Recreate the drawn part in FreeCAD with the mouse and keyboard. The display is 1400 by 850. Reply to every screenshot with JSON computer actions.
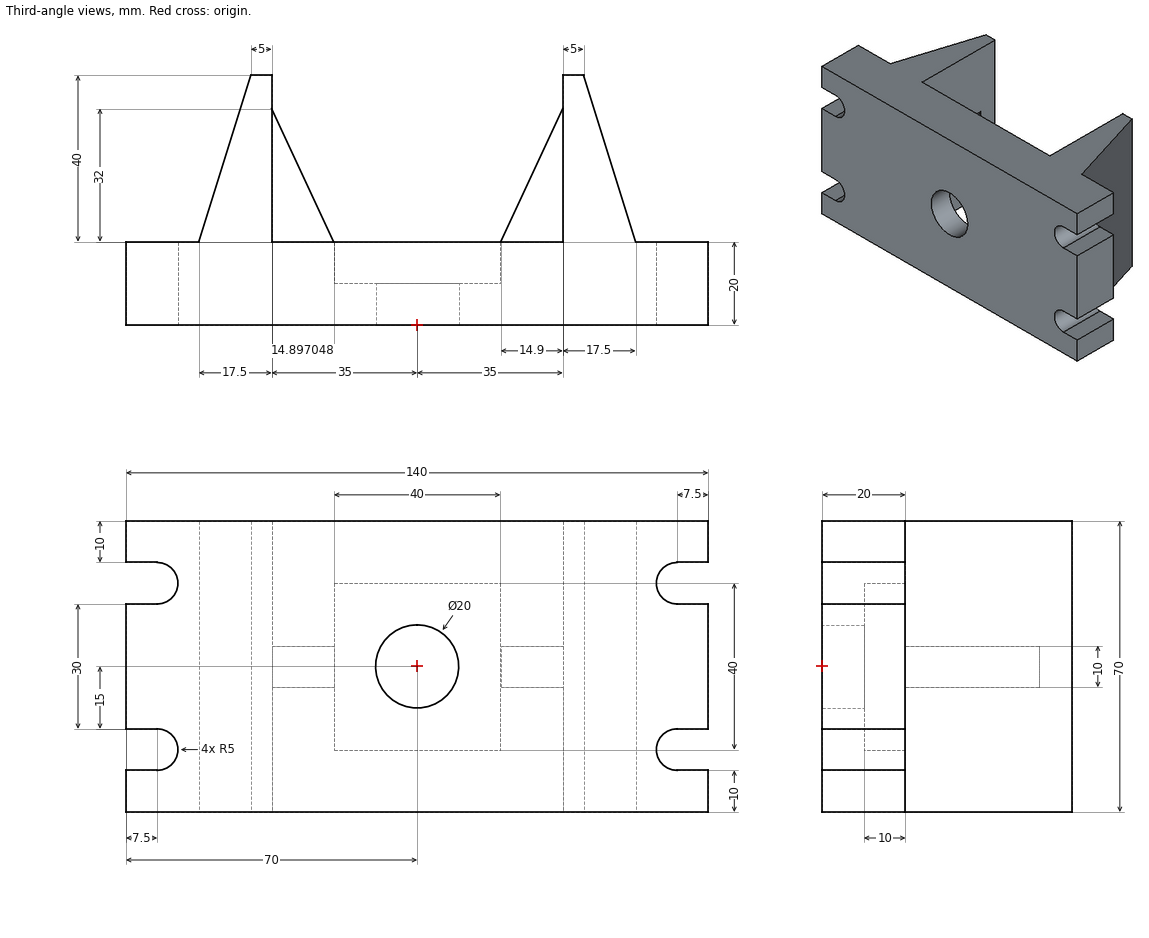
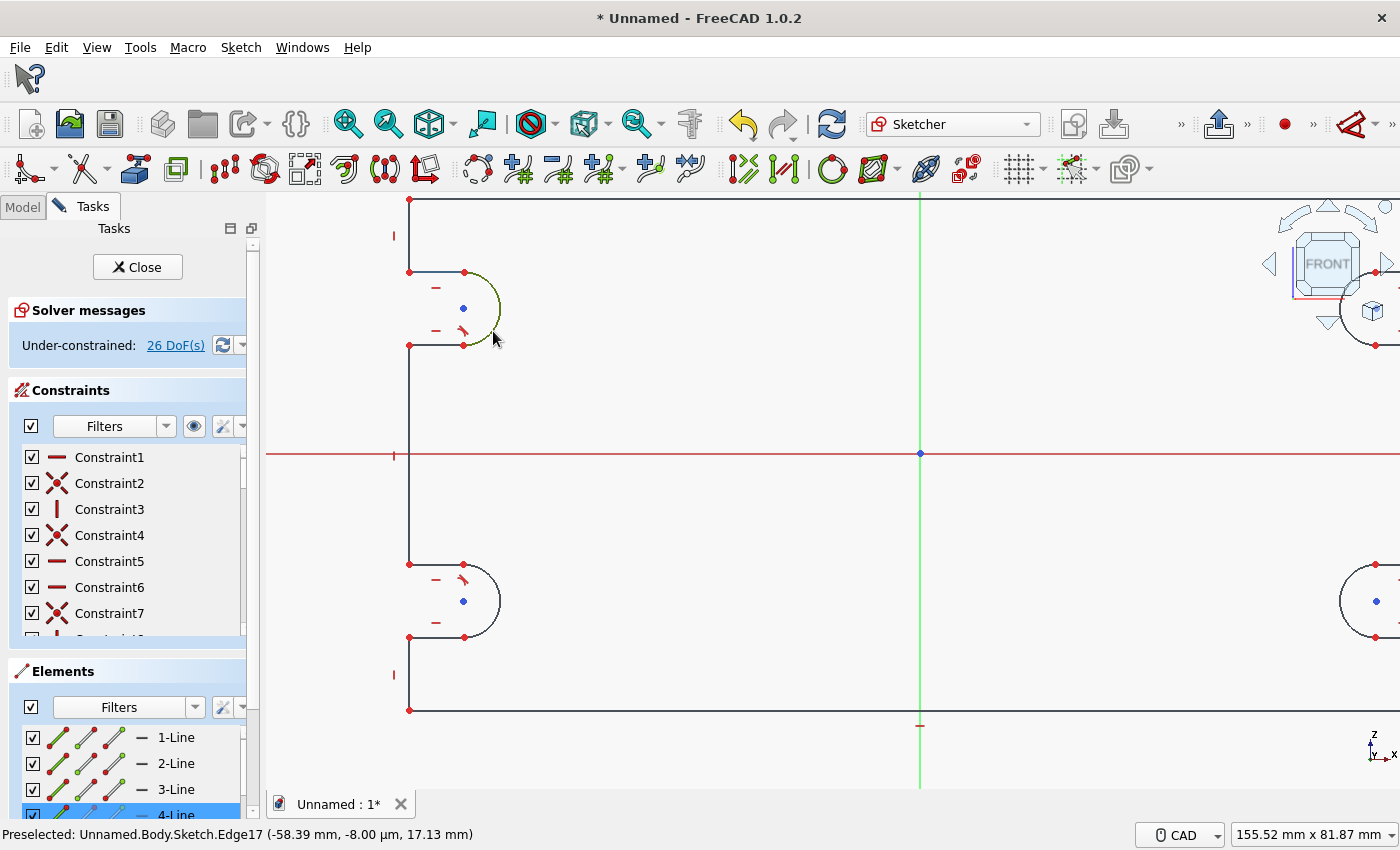
{"action": "key", "text": "t"}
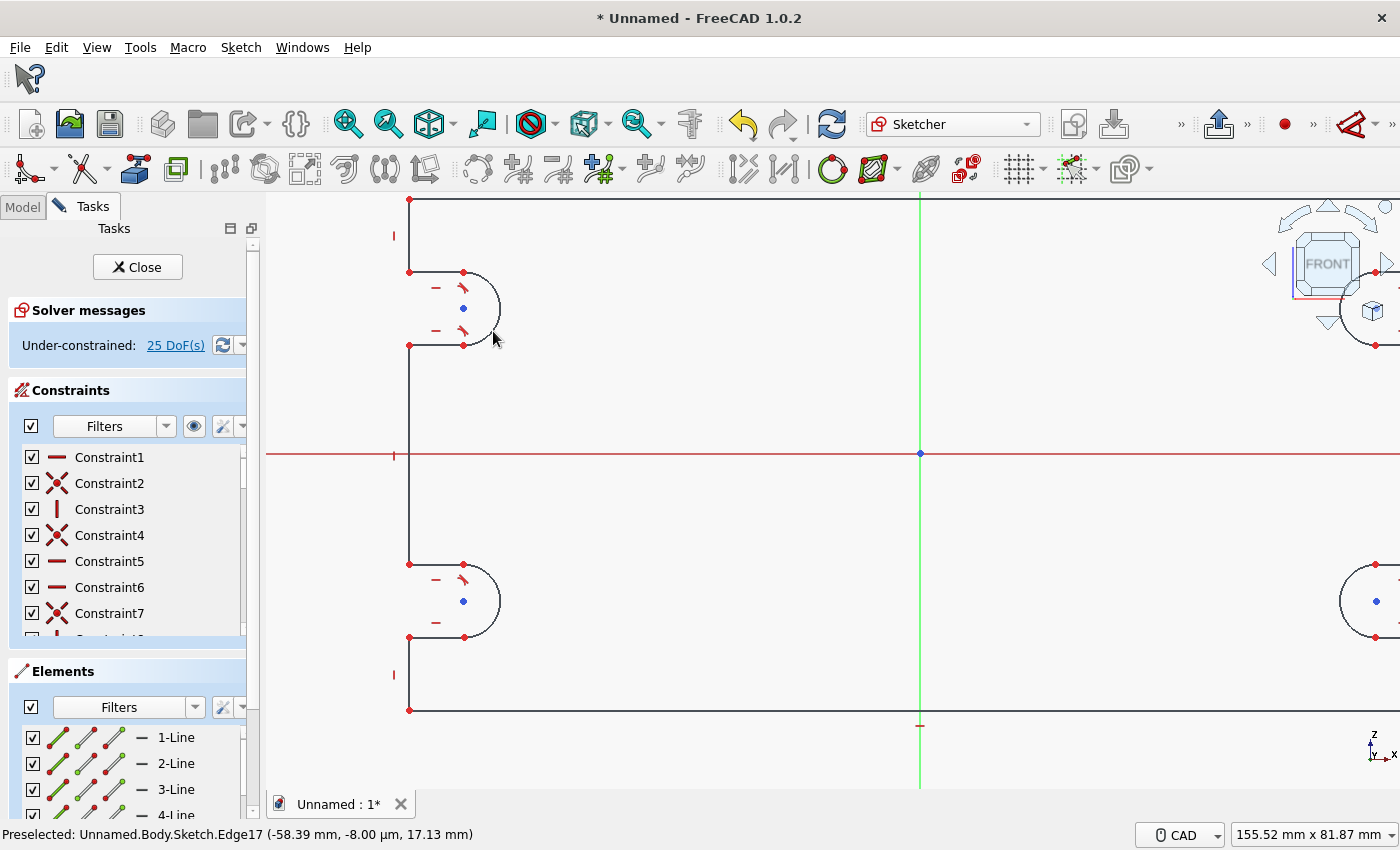
{"action": "scroll", "coordinate": [448, 566], "scroll_direction": "down", "scroll_amount": 2}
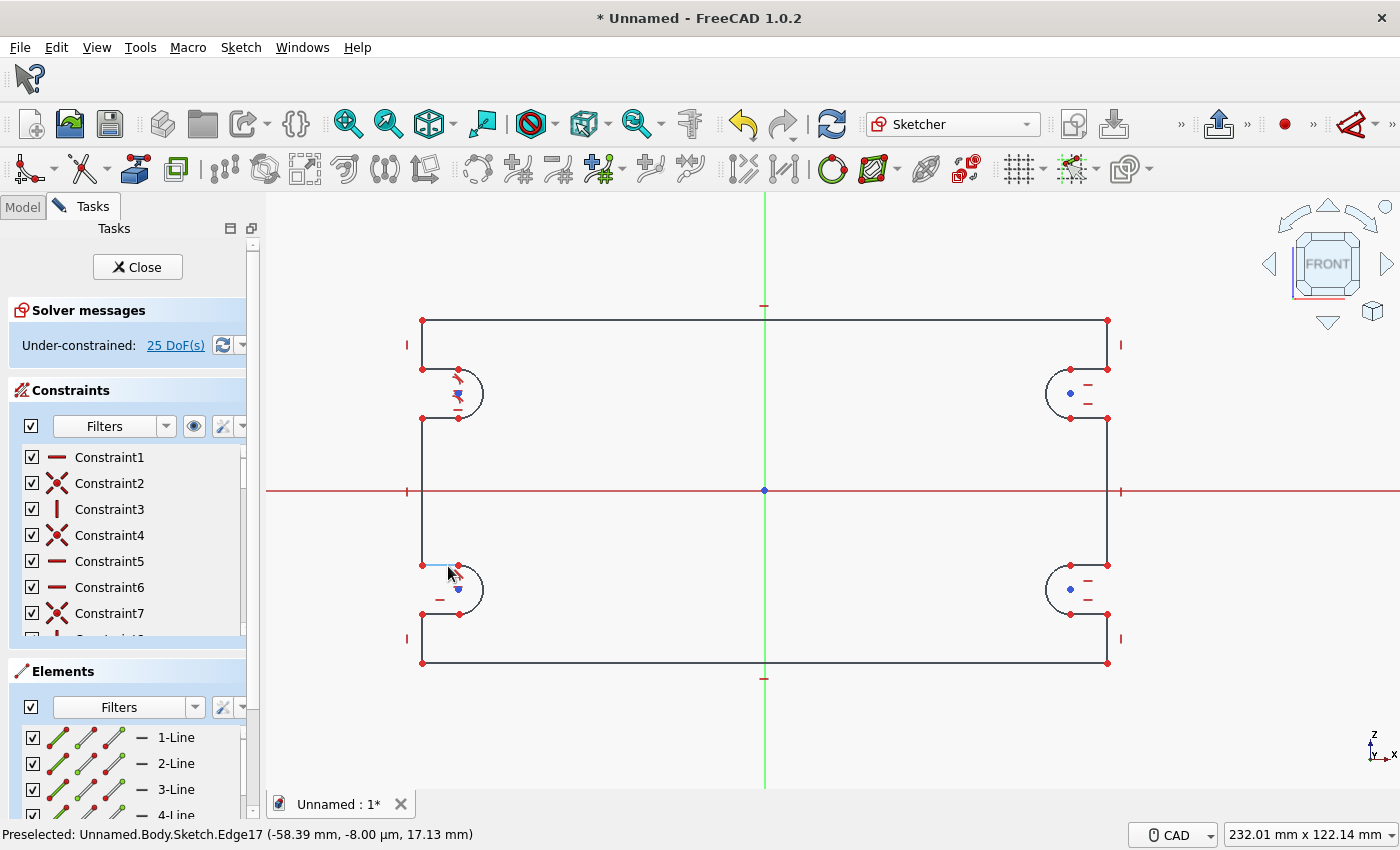
{"action": "scroll", "coordinate": [1096, 369], "scroll_direction": "up", "scroll_amount": 2}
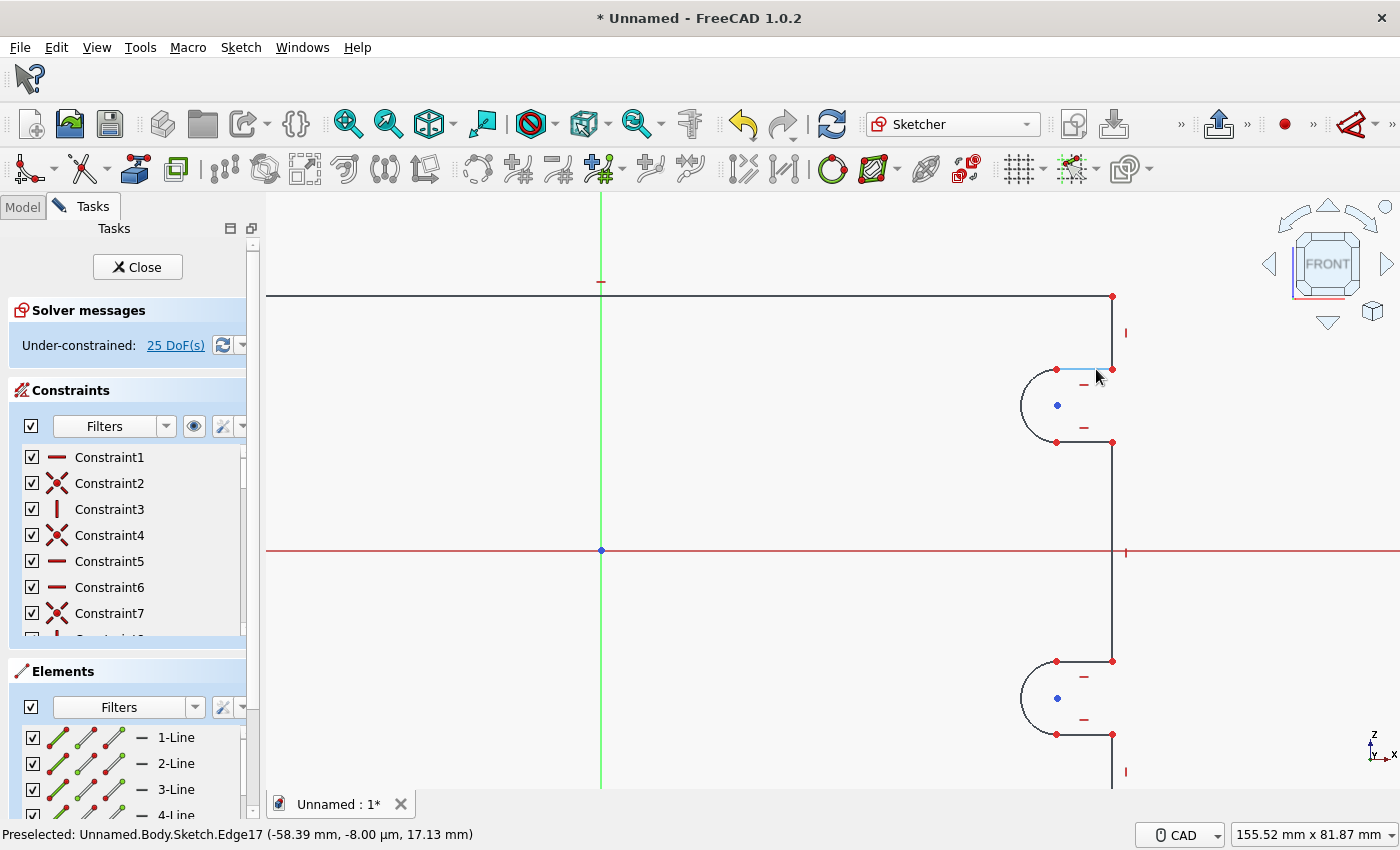
{"action": "left_click", "coordinate": [1095, 369]}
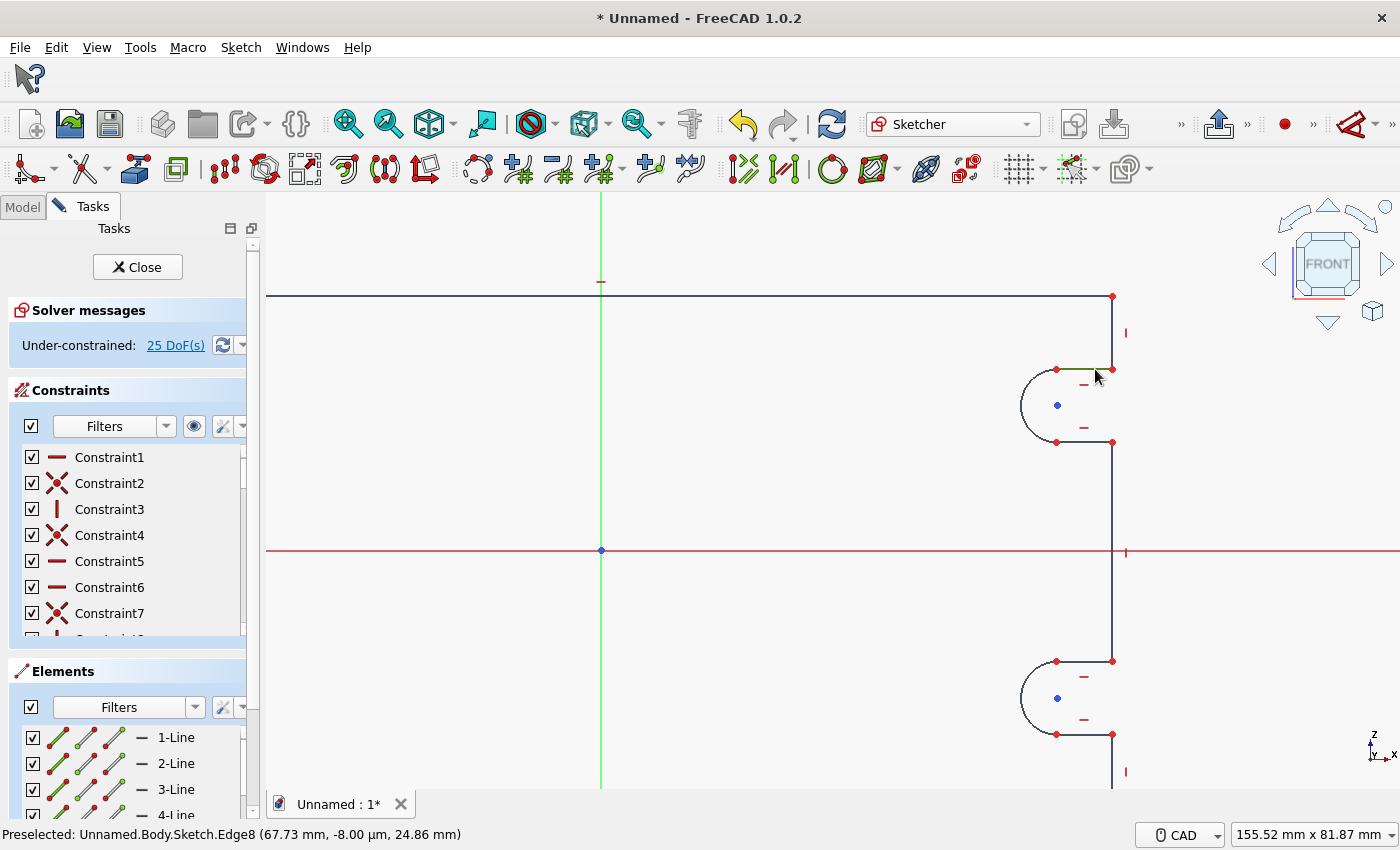
{"action": "left_click", "coordinate": [1028, 385]}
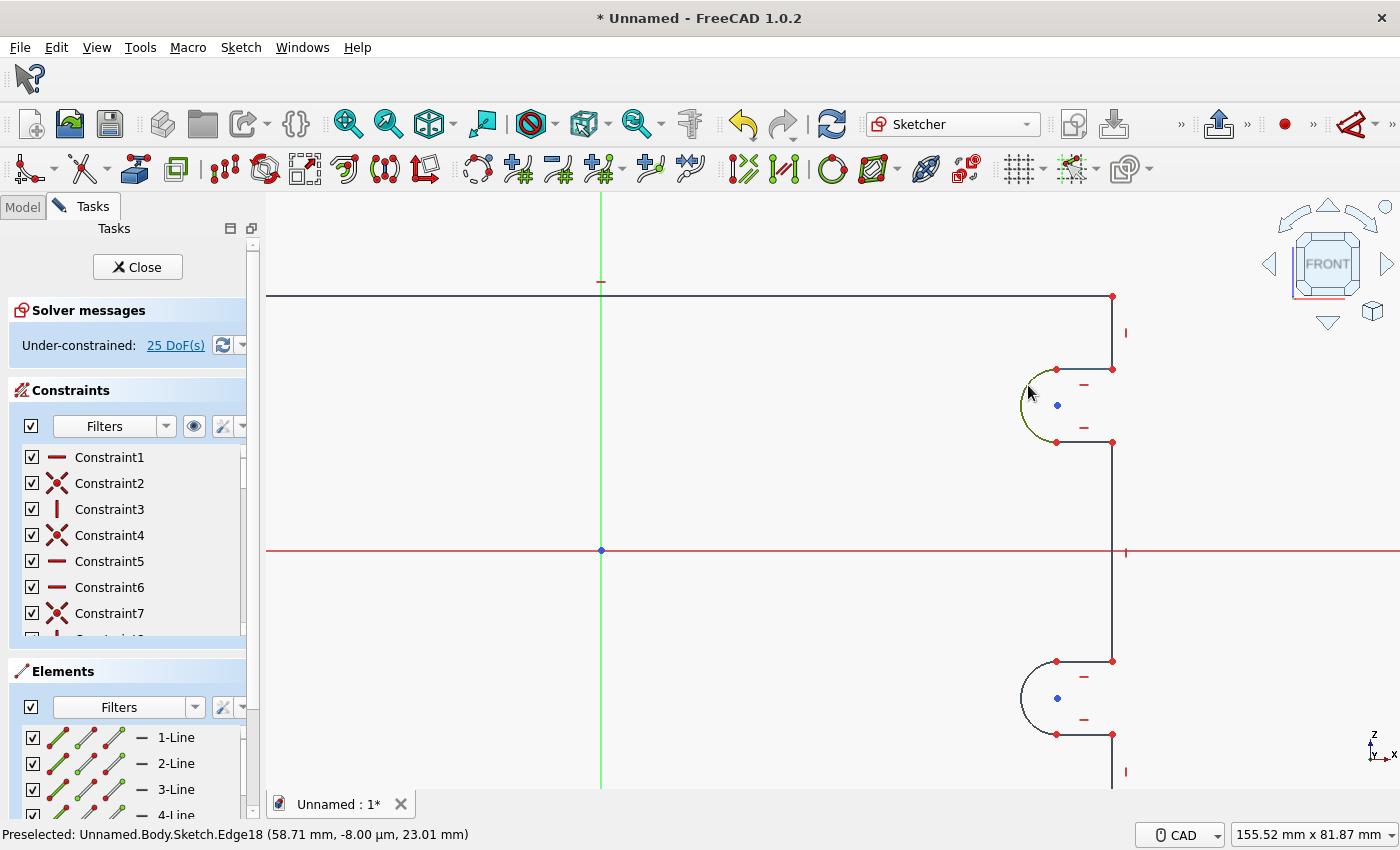
{"action": "key", "text": "t"}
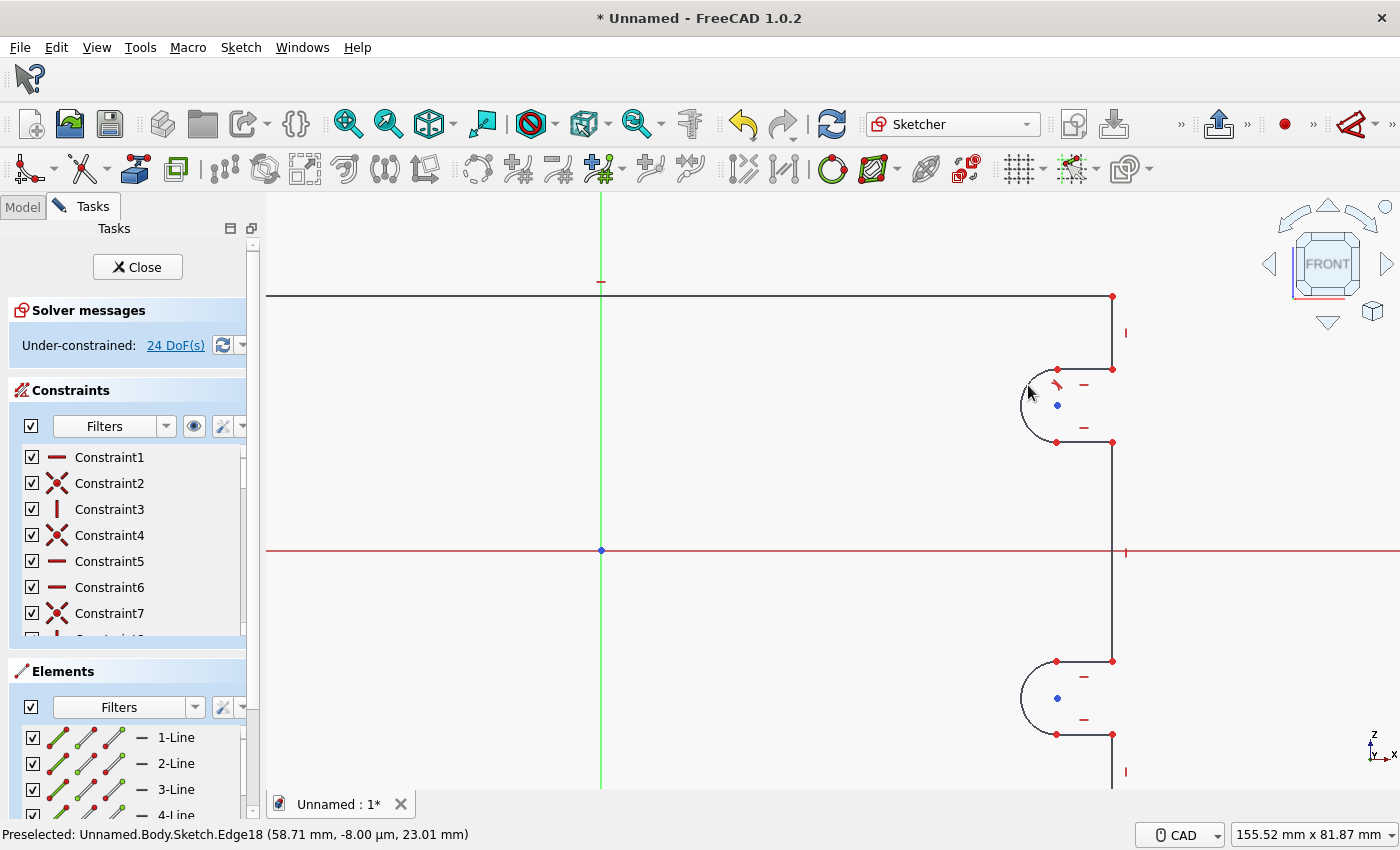
{"action": "left_click", "coordinate": [1073, 442]}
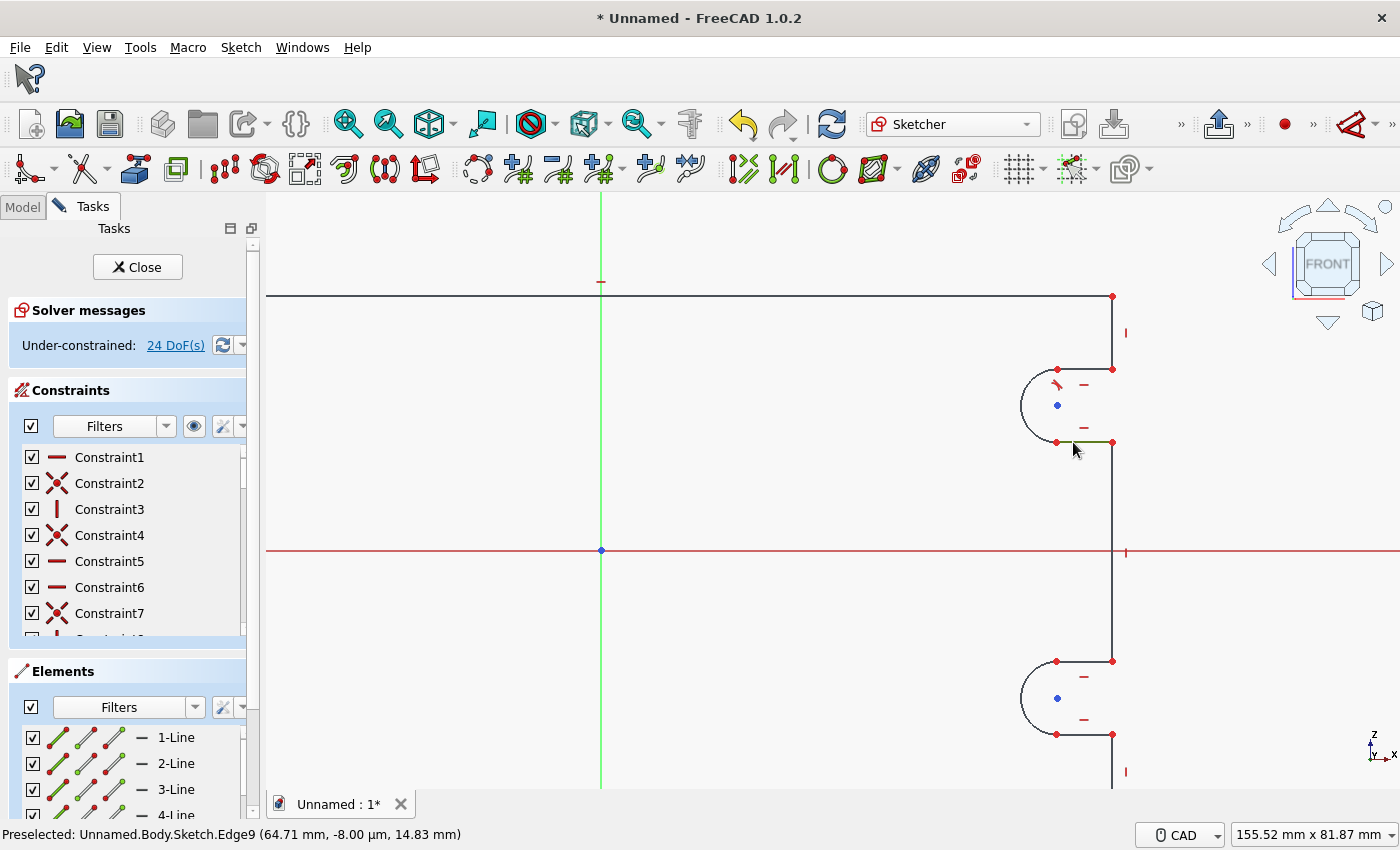
{"action": "left_click", "coordinate": [1028, 384]}